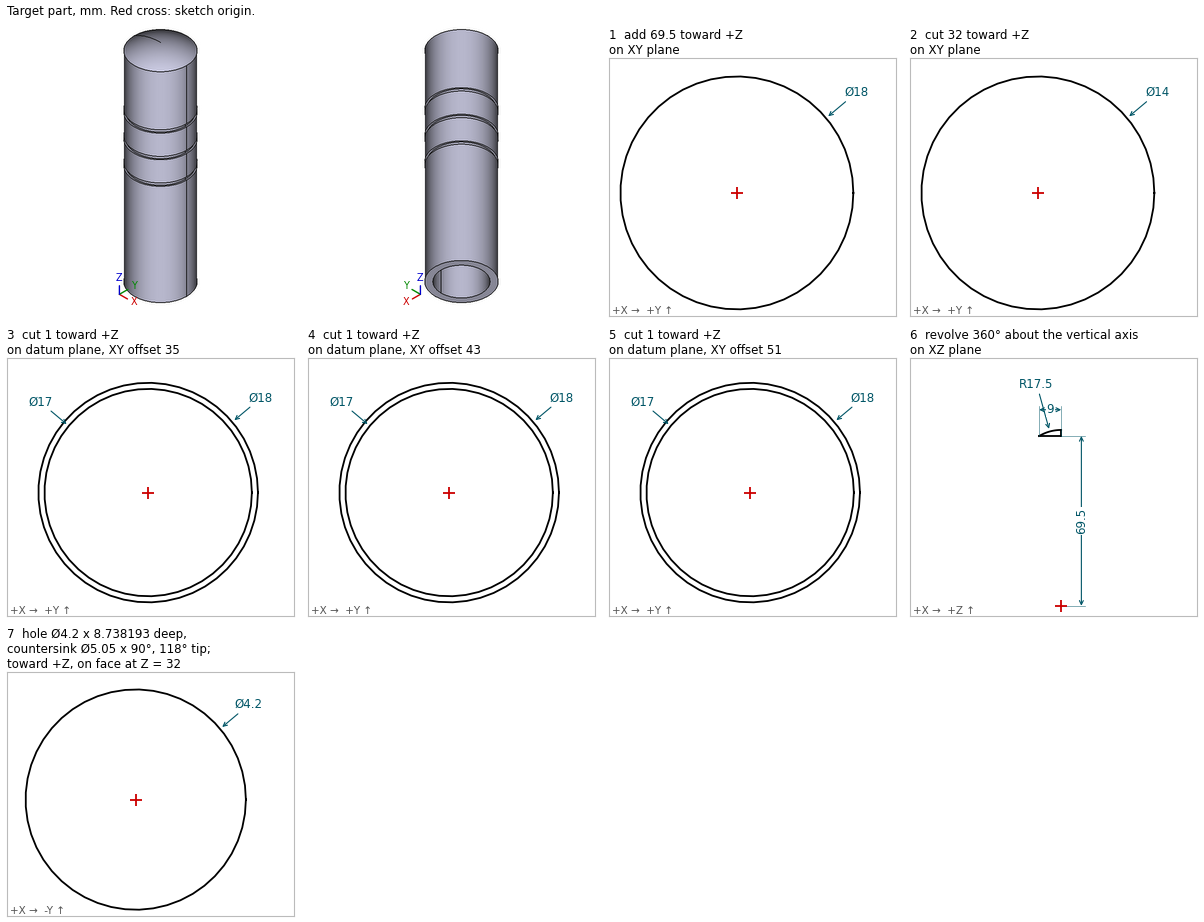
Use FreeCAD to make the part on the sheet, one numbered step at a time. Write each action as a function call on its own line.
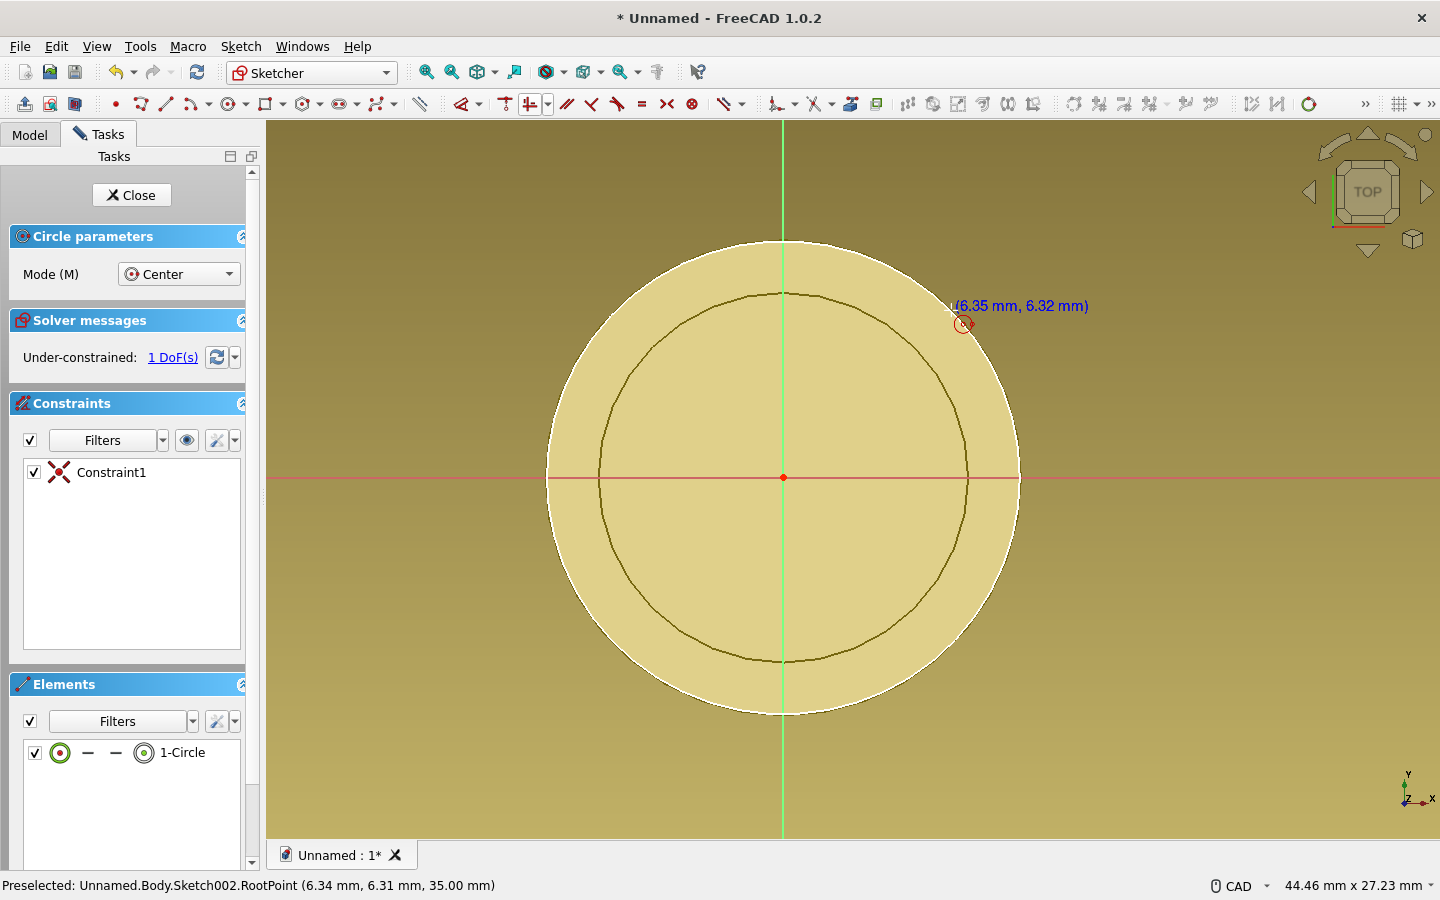
click(783, 478)
click(942, 319)
key(Escape)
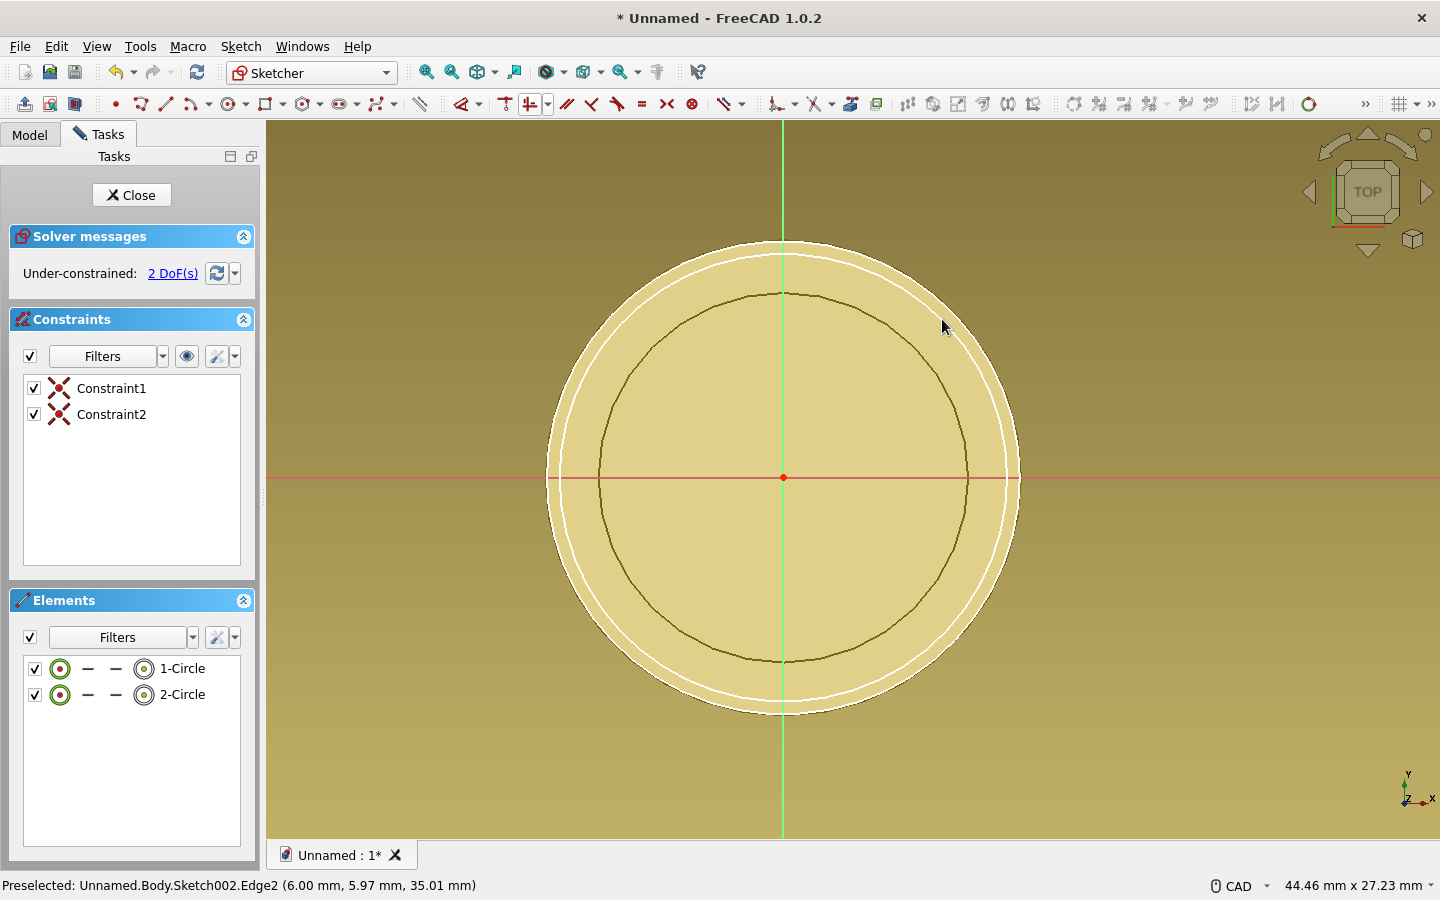
key(d)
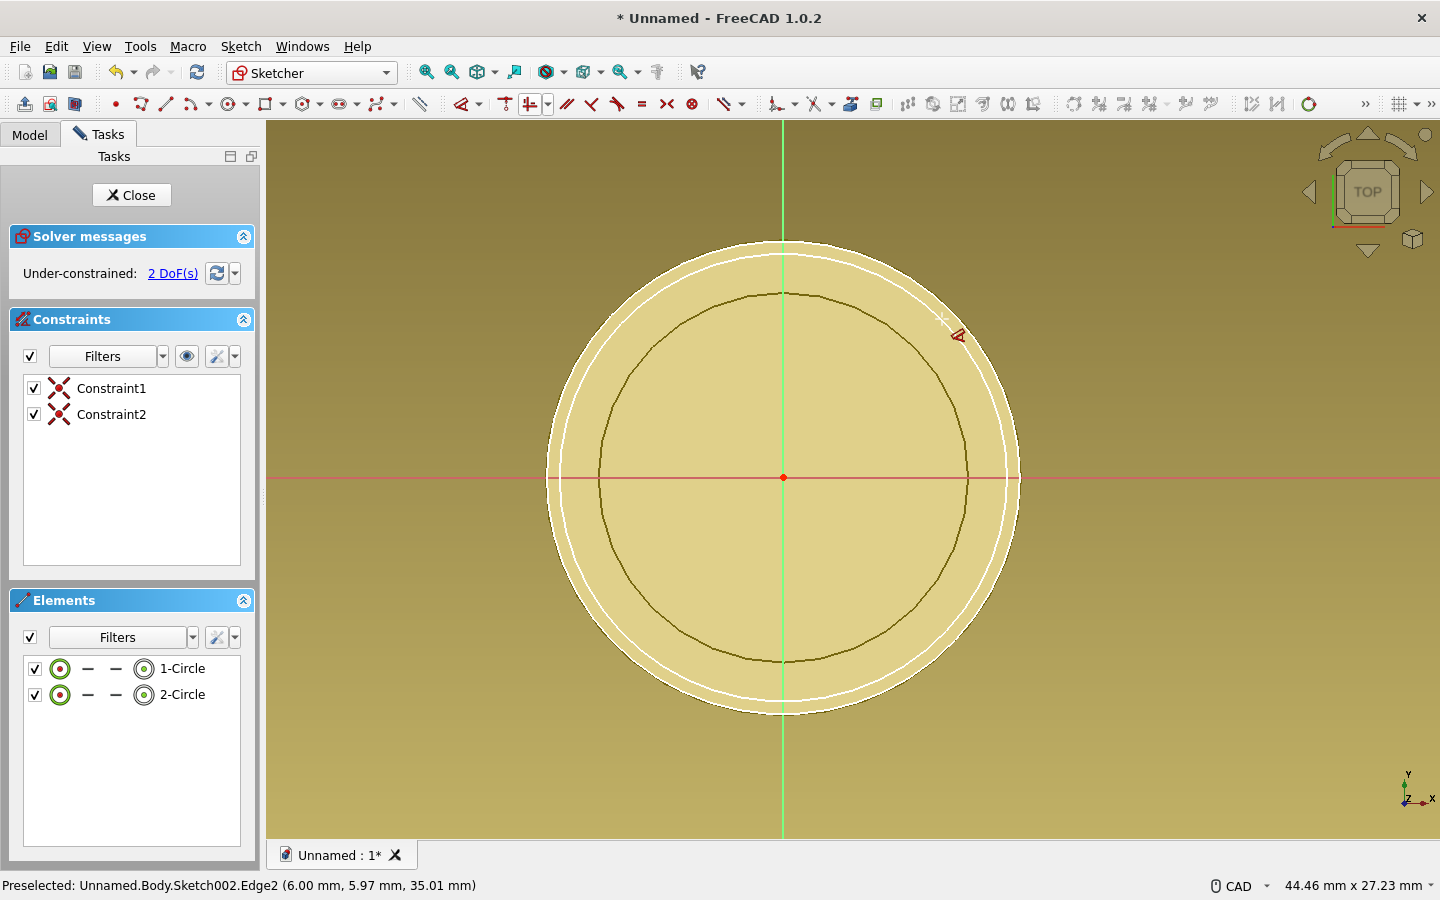
click(950, 310)
click(973, 287)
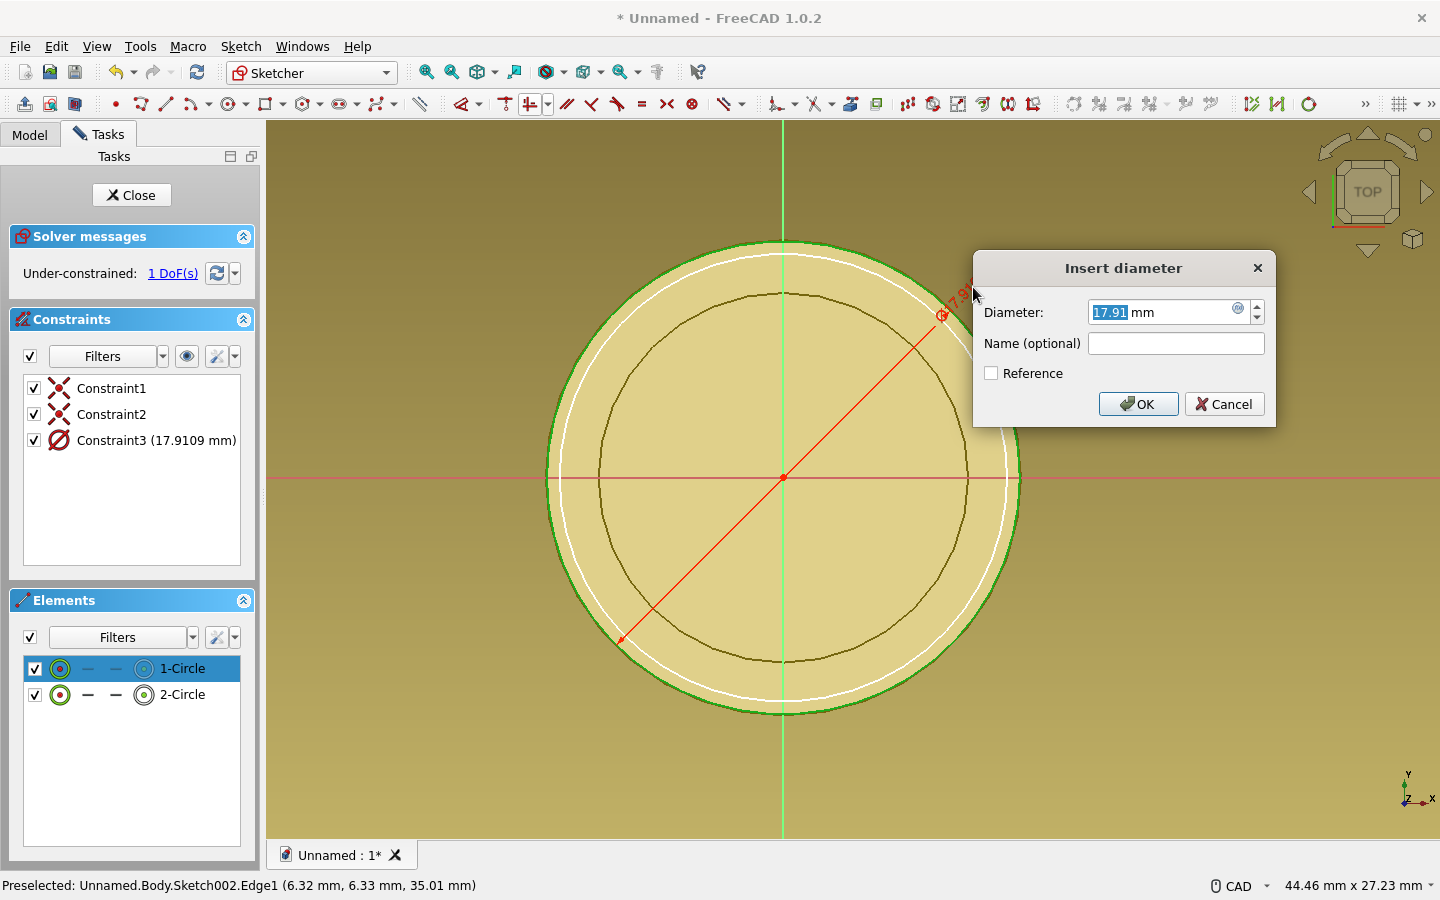
text(18)
key(Return)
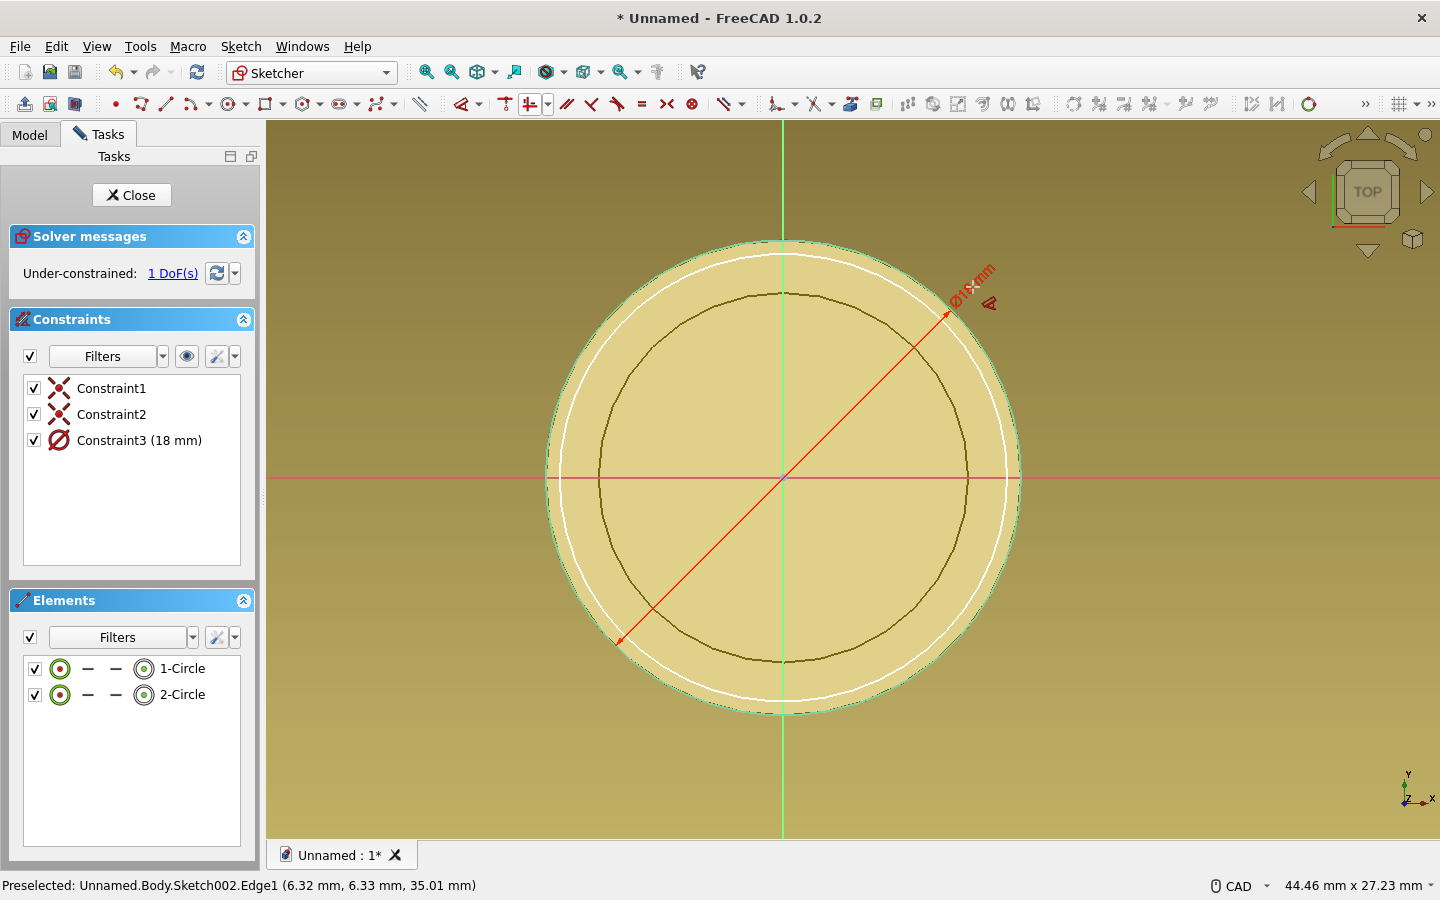
click(941, 319)
click(1028, 405)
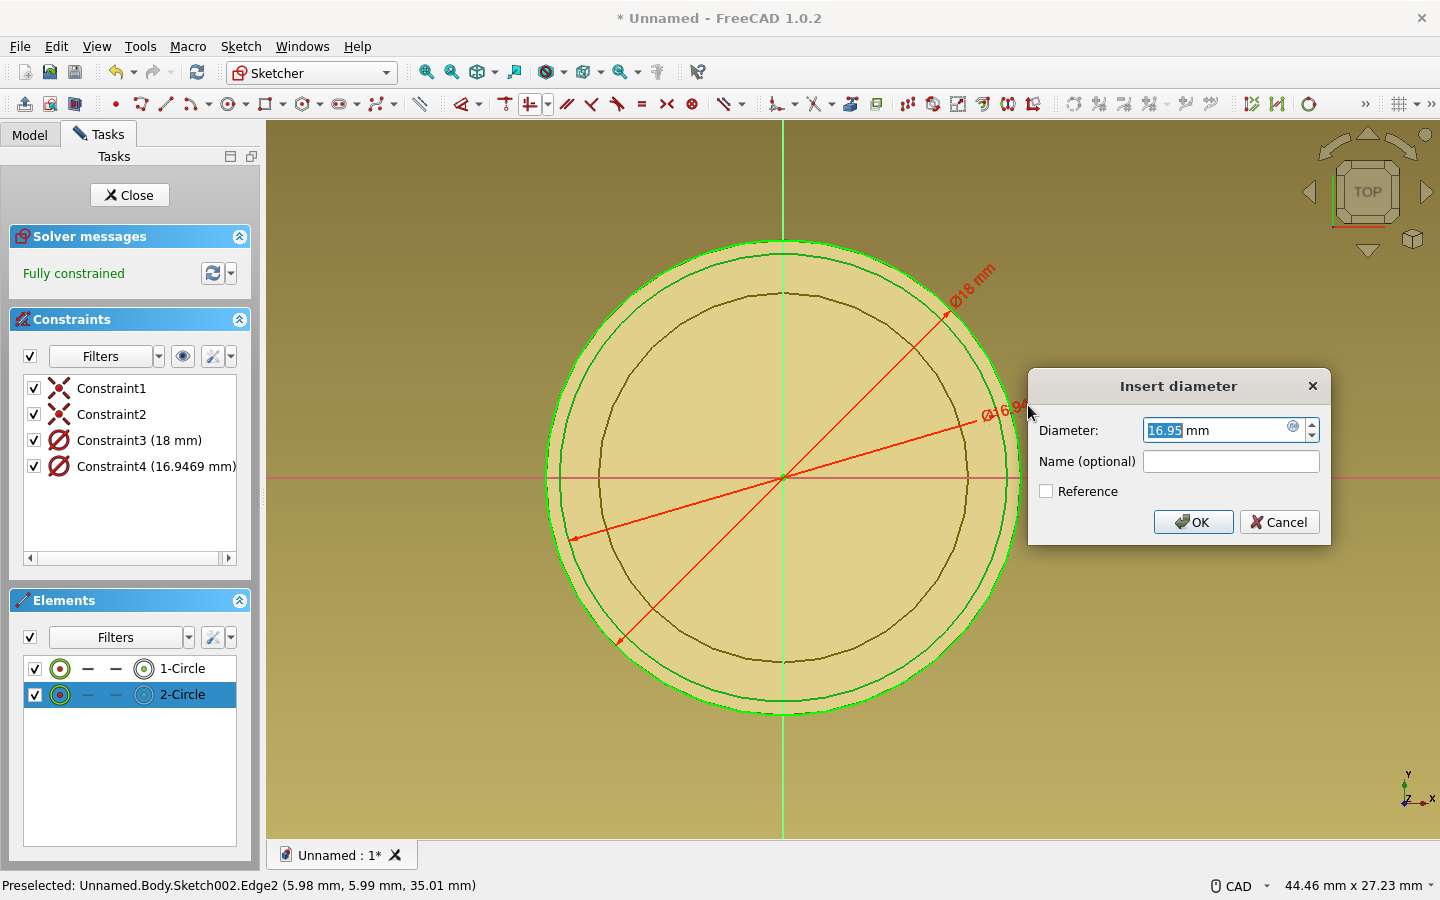
text(17)
key(Return)
key(Escape)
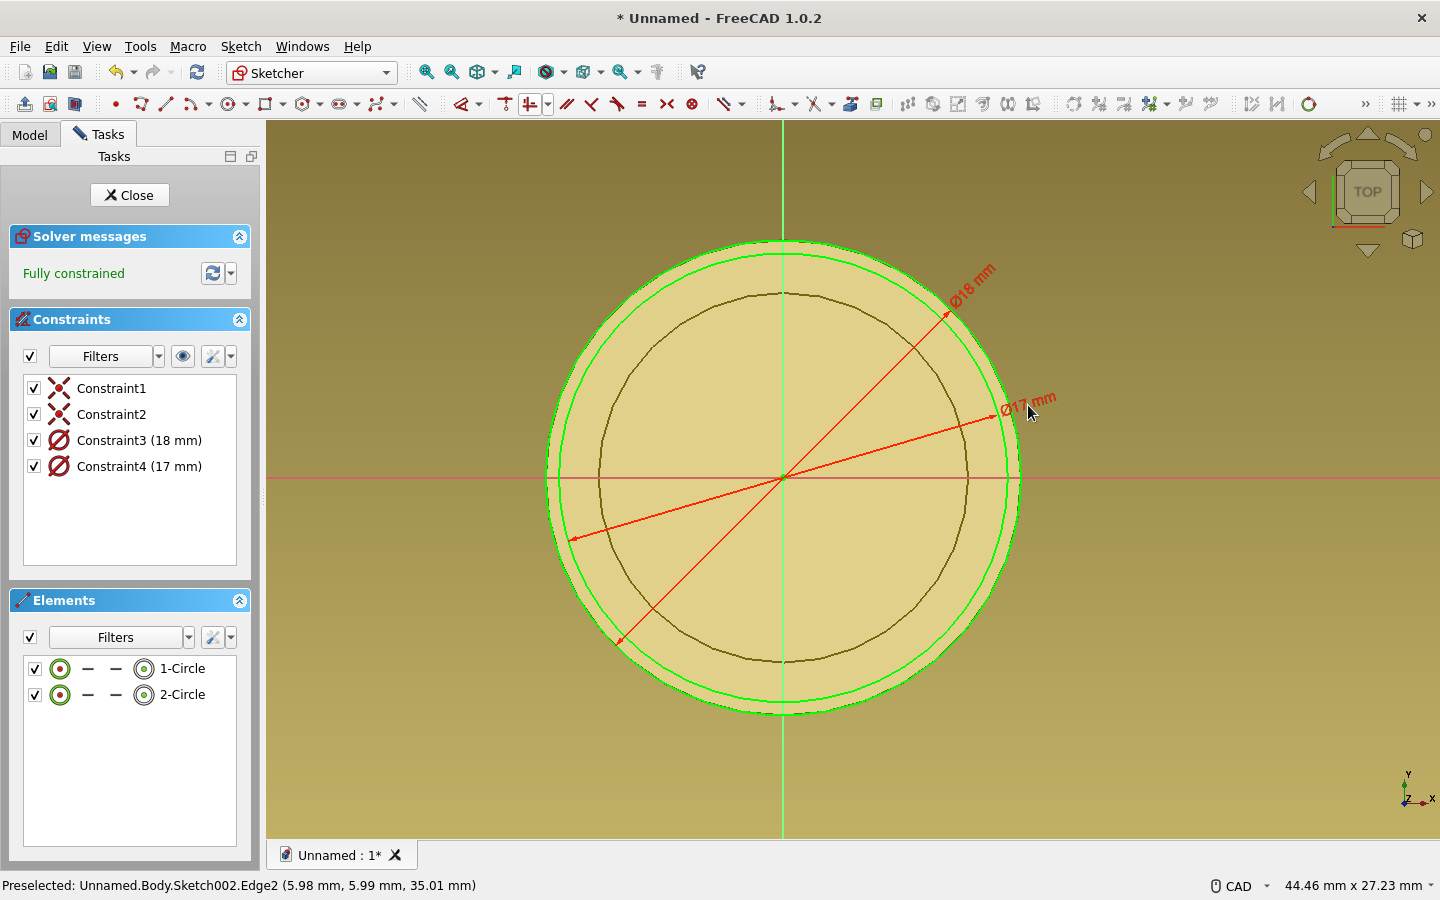
click(130, 195)